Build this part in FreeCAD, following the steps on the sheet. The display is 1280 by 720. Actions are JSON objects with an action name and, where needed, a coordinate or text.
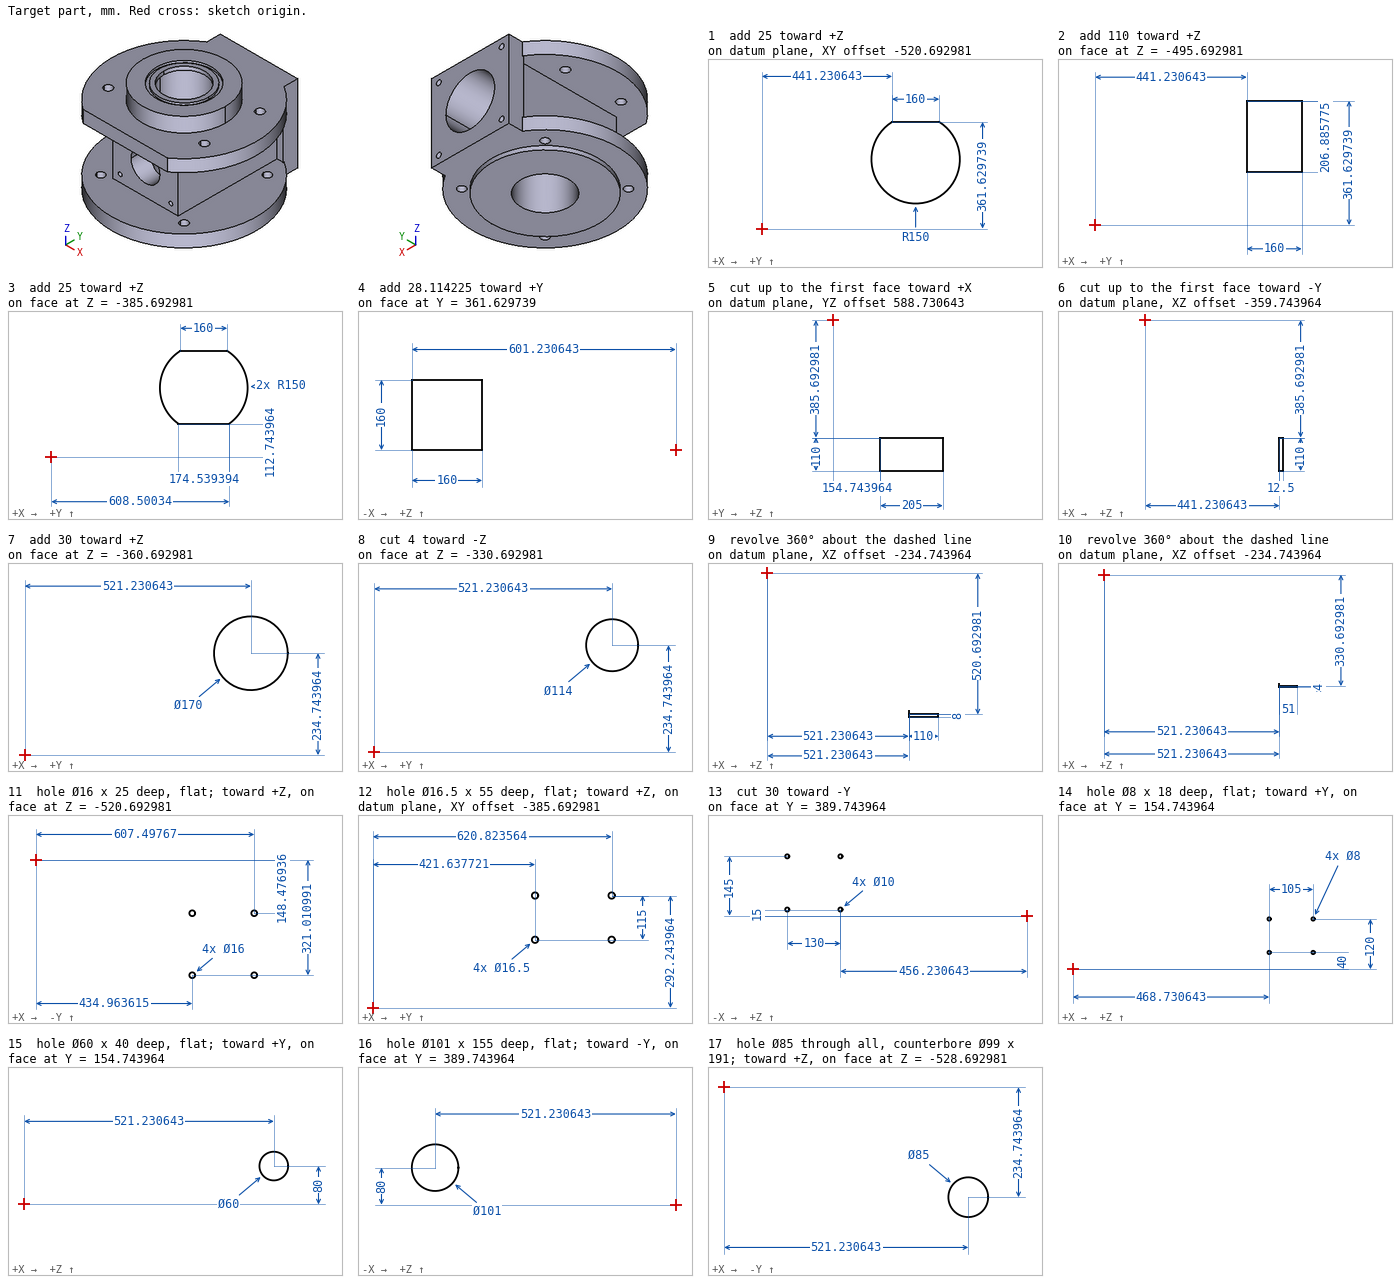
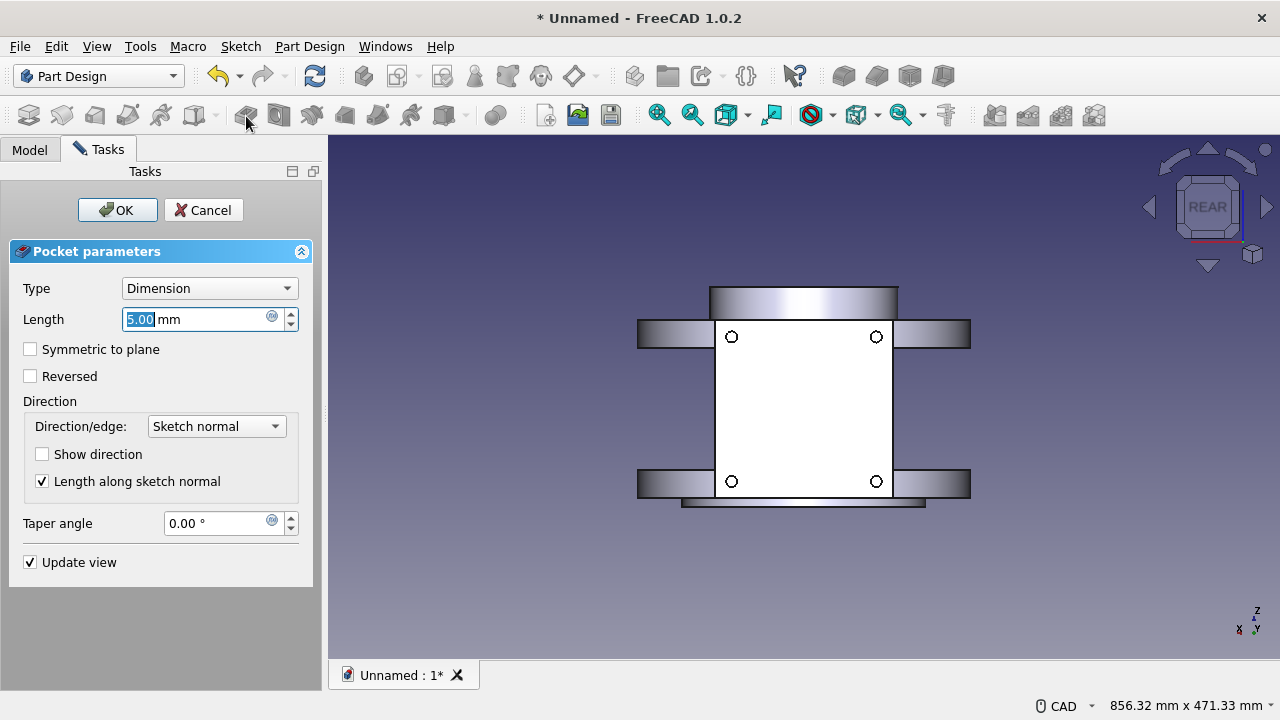
{"action": "type", "text": "30"}
{"action": "key", "text": "Tab"}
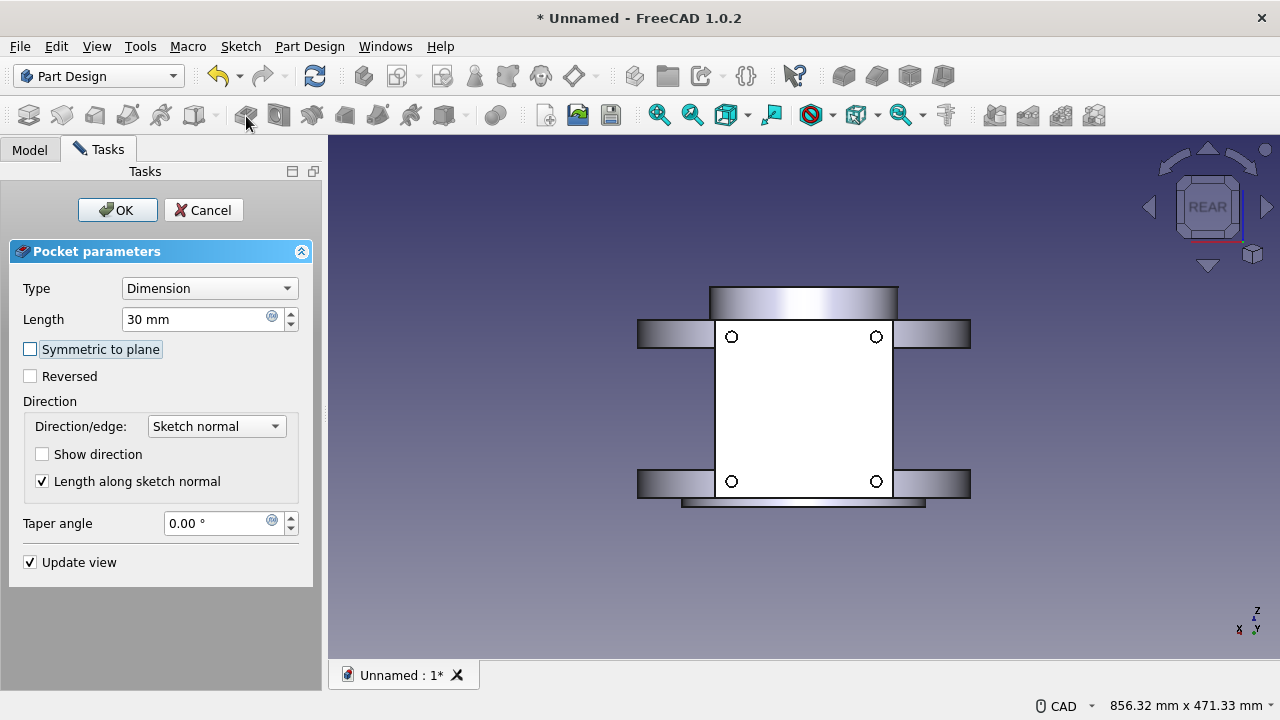
{"action": "left_click", "coordinate": [118, 210]}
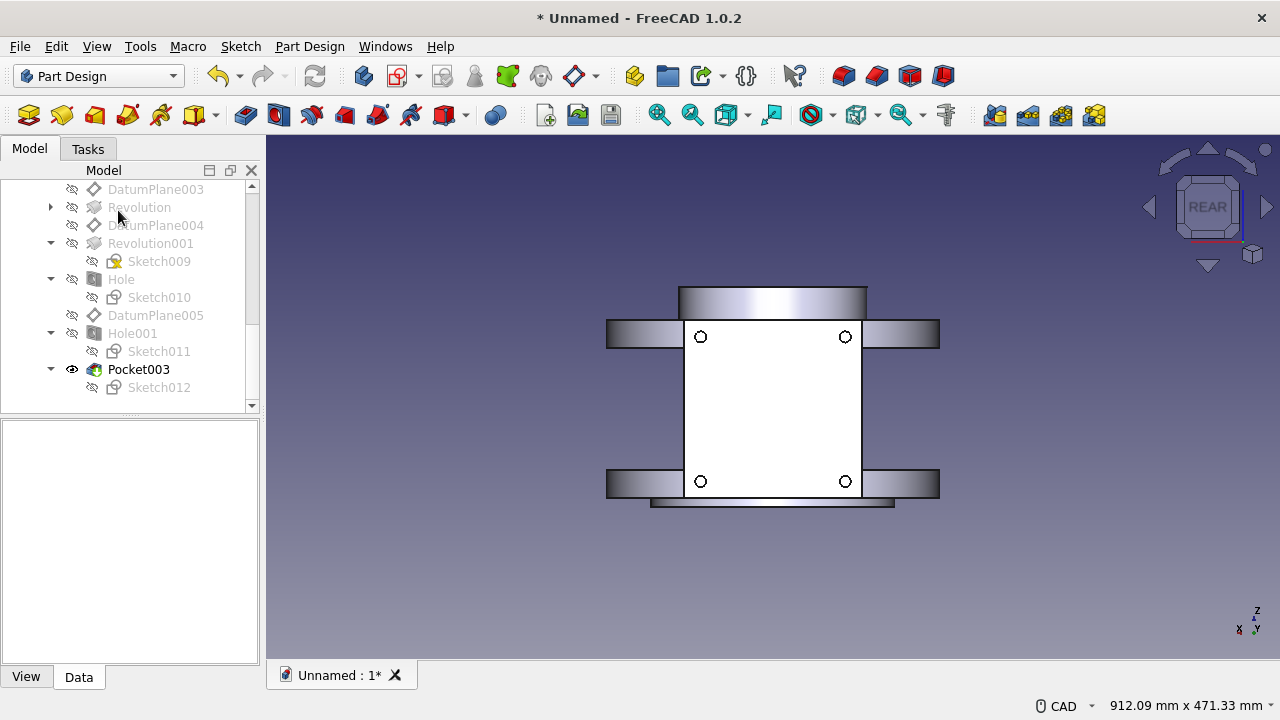
{"action": "left_click", "coordinate": [660, 116]}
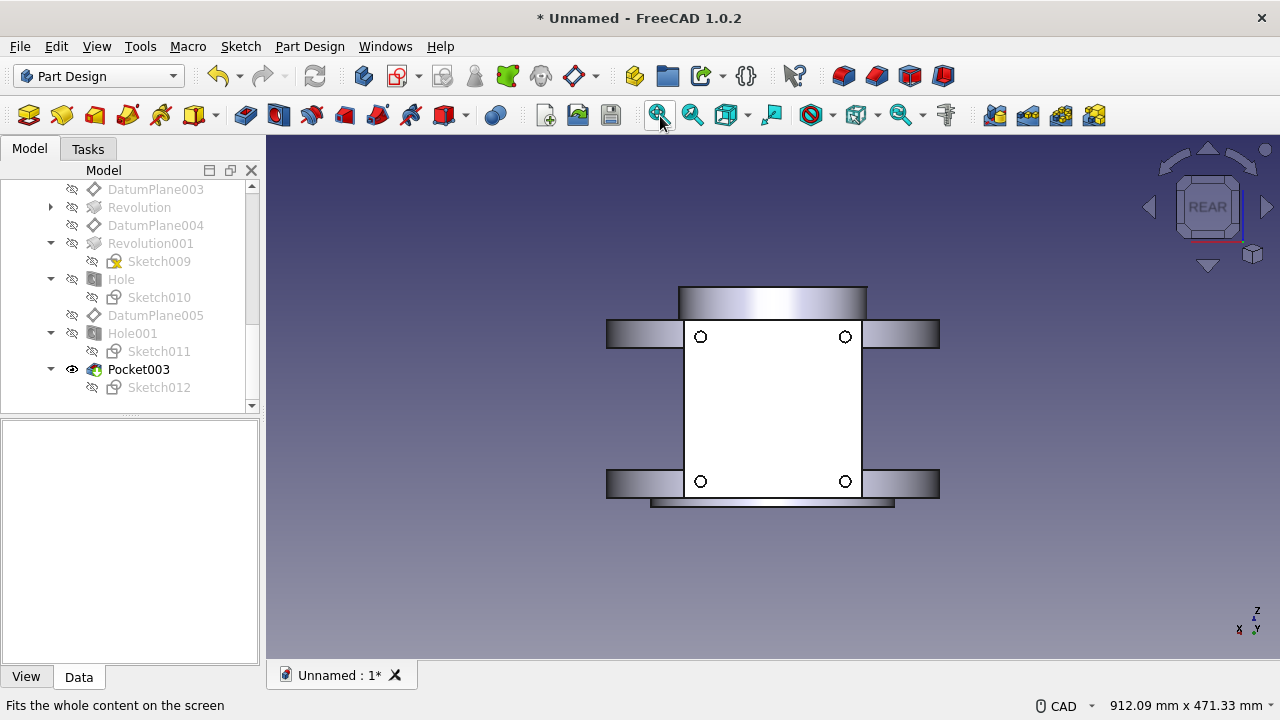
{"action": "key", "text": "0"}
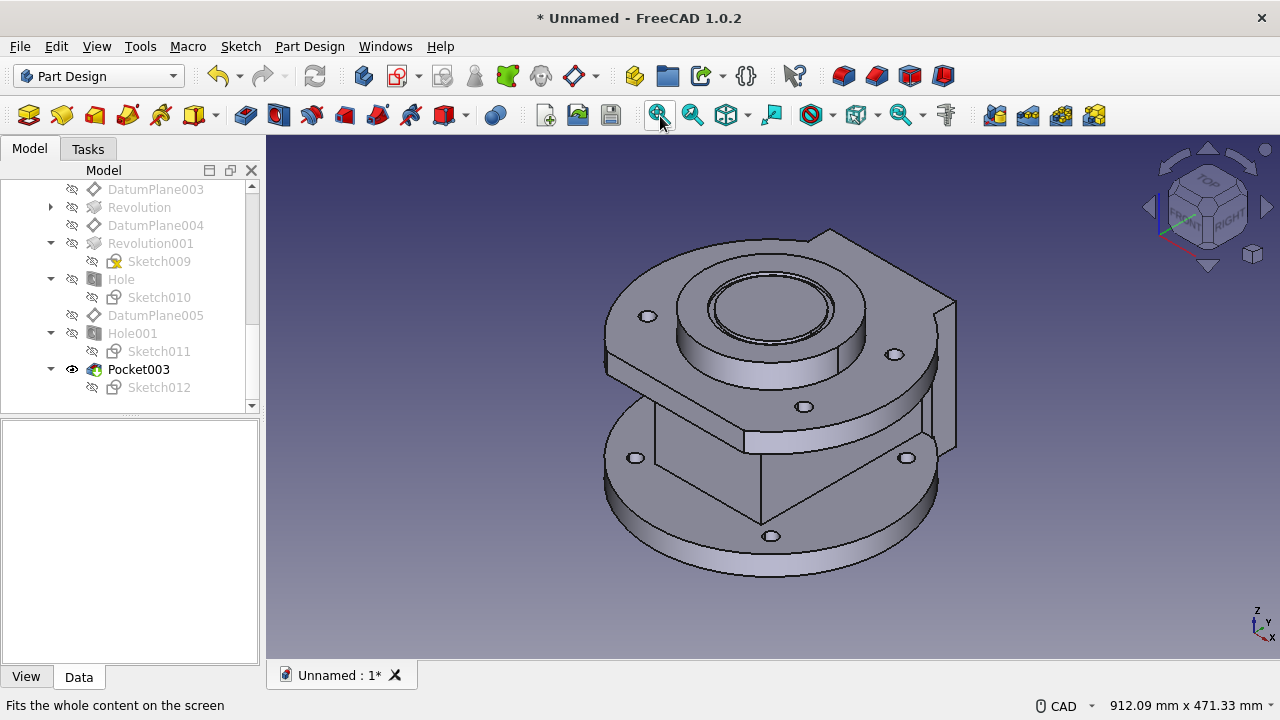
{"action": "left_click", "coordinate": [708, 443]}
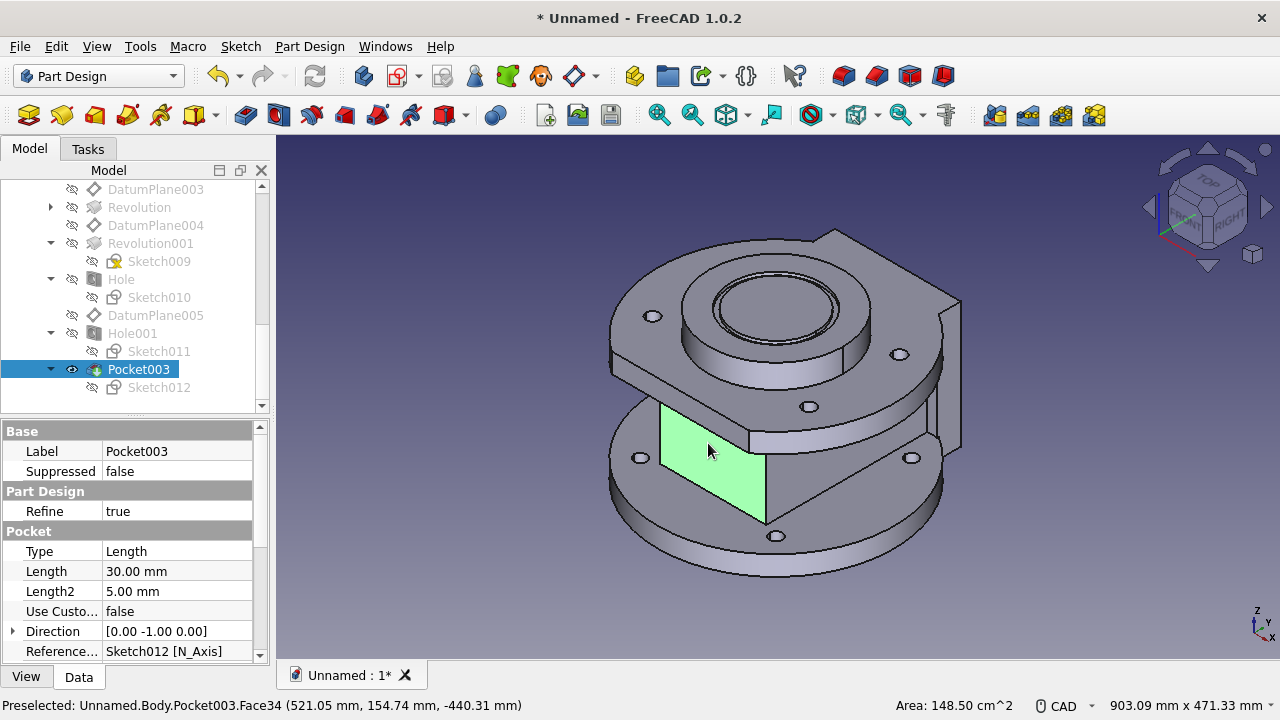
{"action": "left_click", "coordinate": [396, 76]}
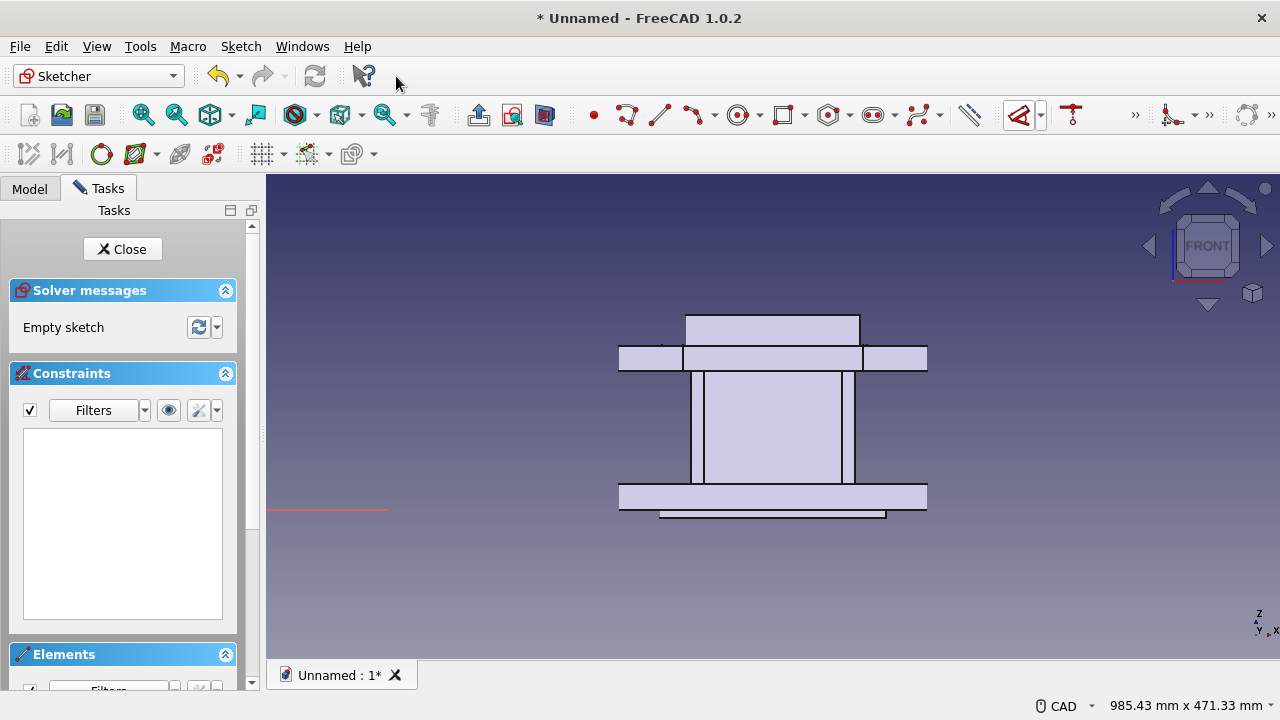
{"action": "scroll", "coordinate": [803, 433], "scroll_direction": "up", "scroll_amount": 6}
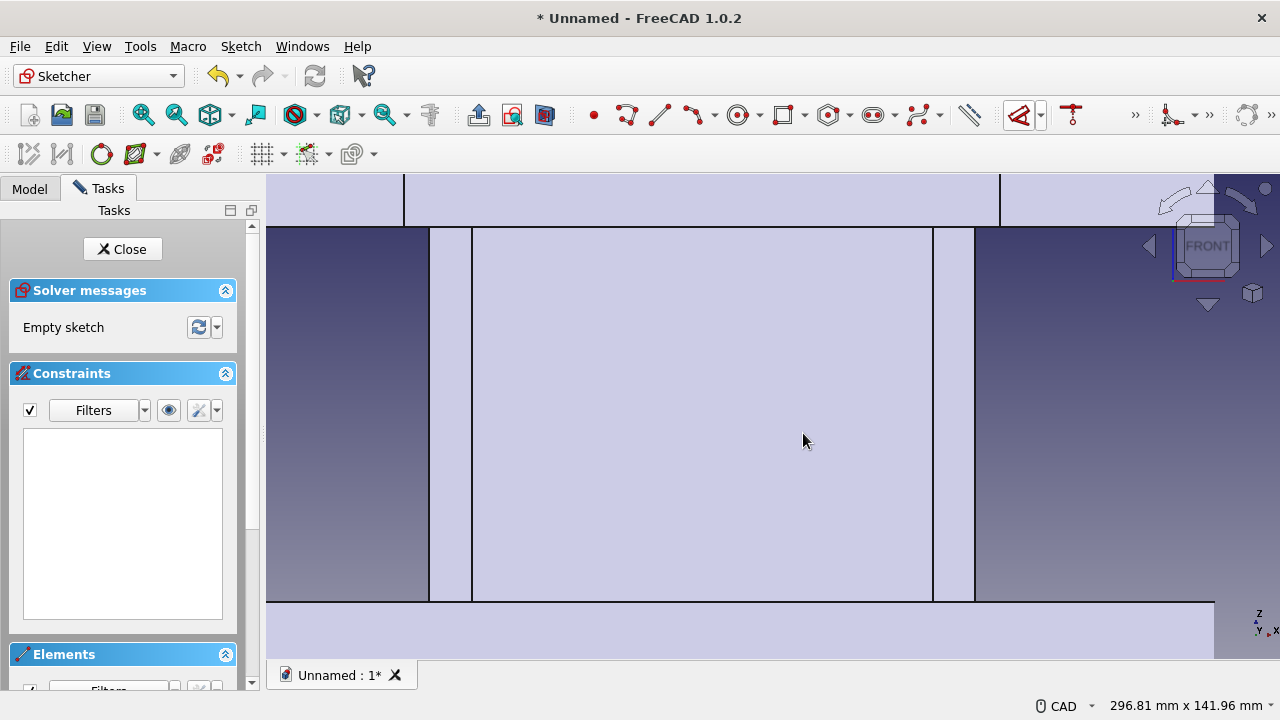
{"action": "left_click", "coordinate": [738, 116]}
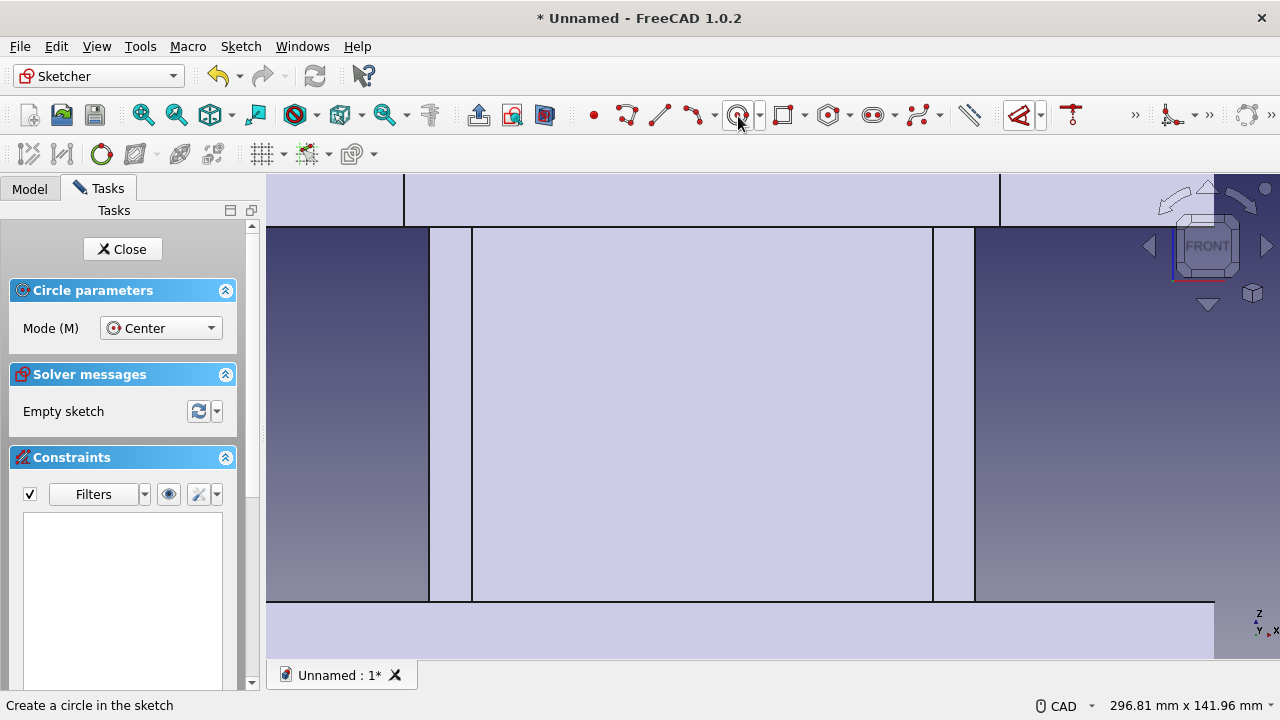
{"action": "scroll", "coordinate": [523, 551], "scroll_direction": "up", "scroll_amount": 3}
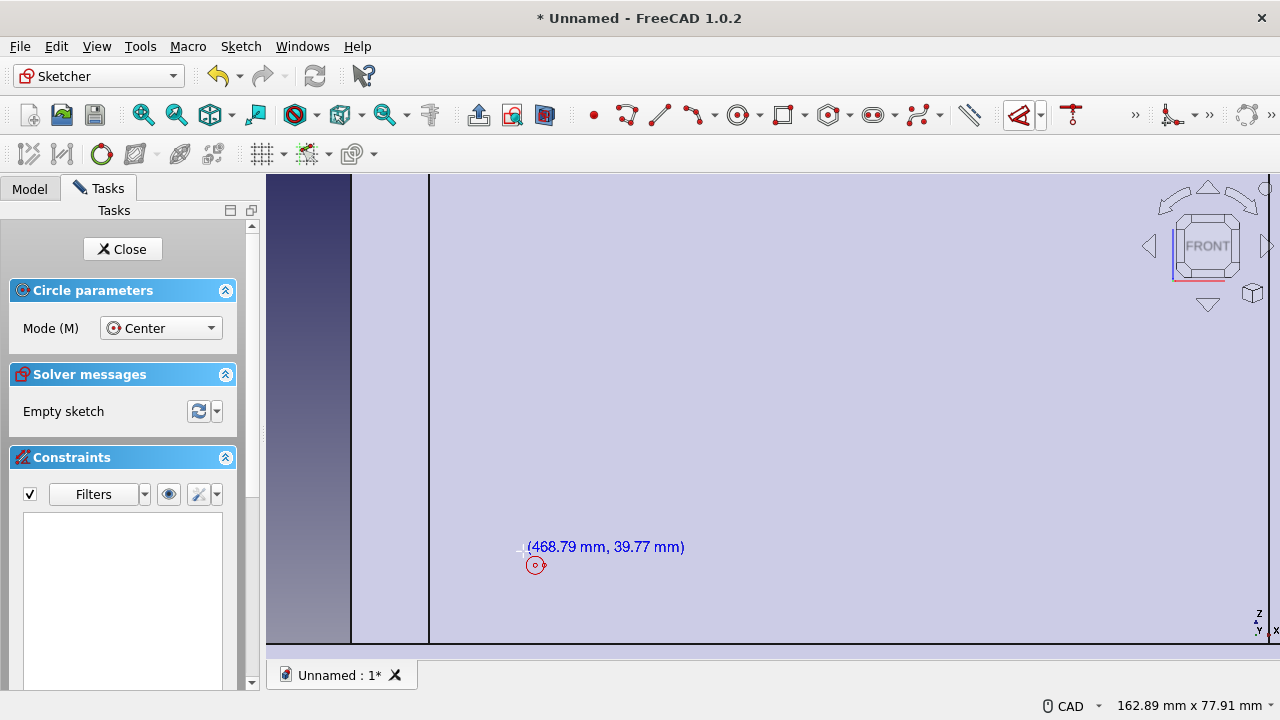
{"action": "left_click", "coordinate": [522, 551]}
{"action": "left_click", "coordinate": [540, 533]}